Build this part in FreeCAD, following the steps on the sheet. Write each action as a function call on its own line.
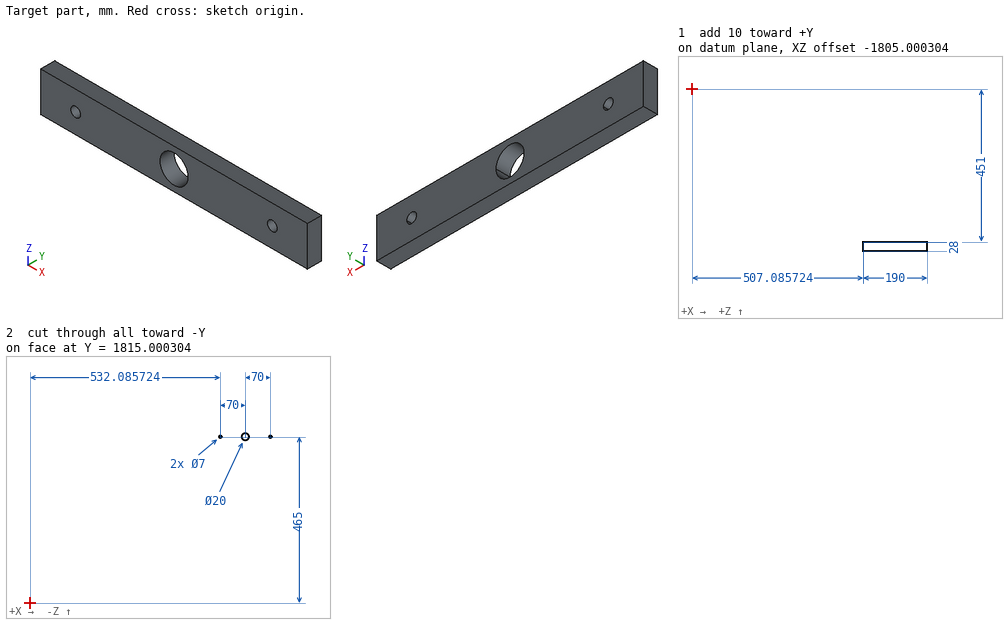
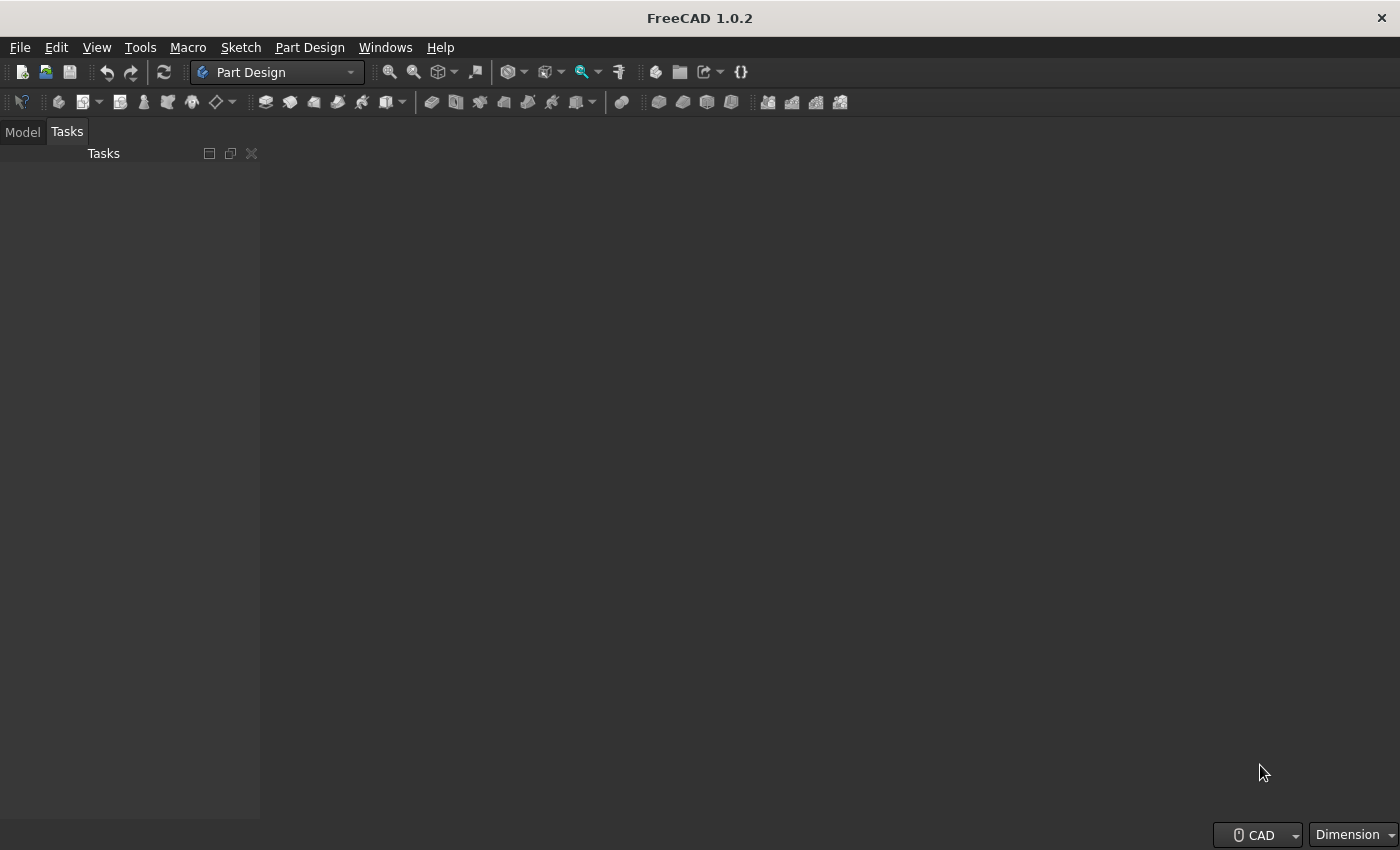
click(22, 72)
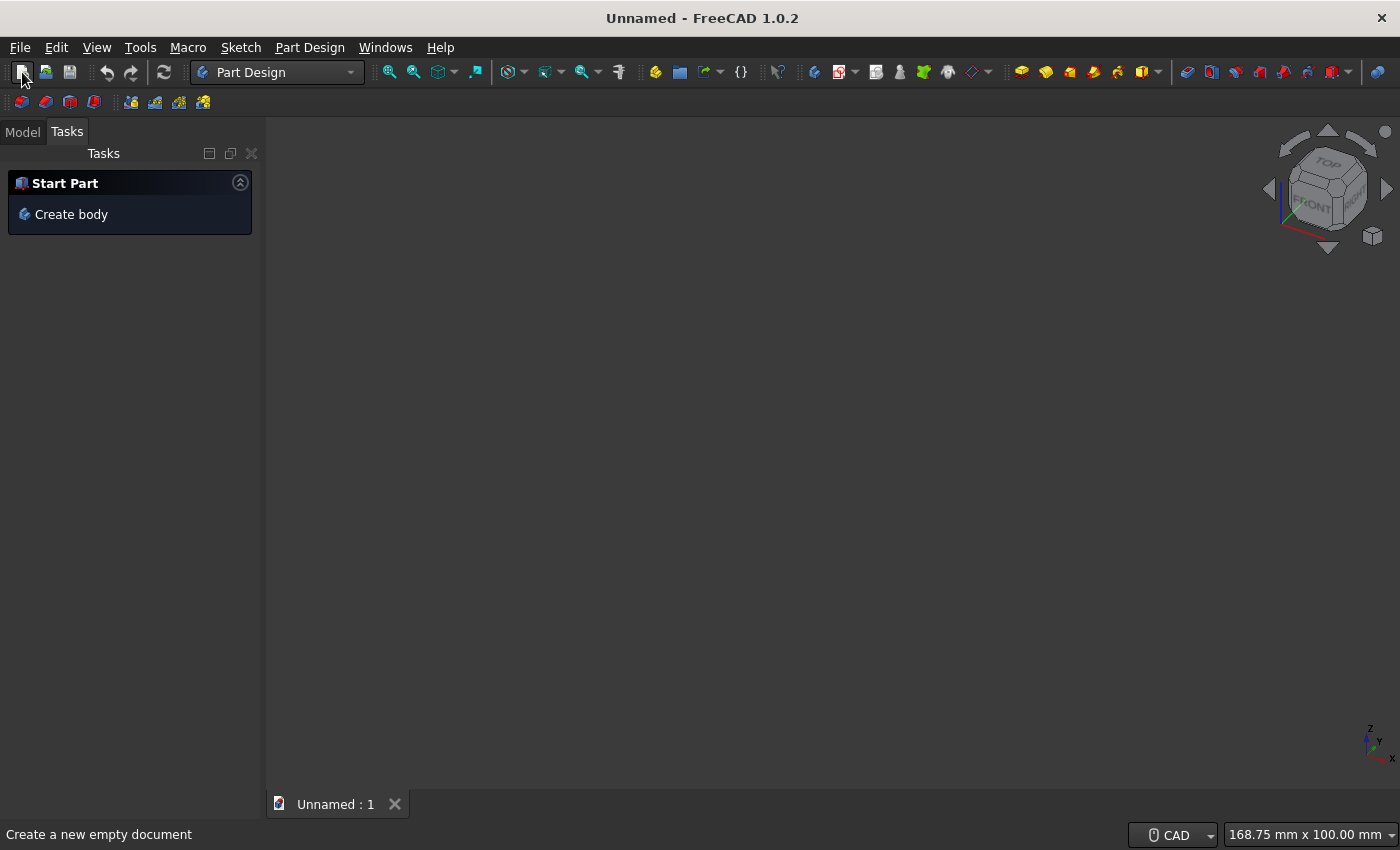
click(816, 72)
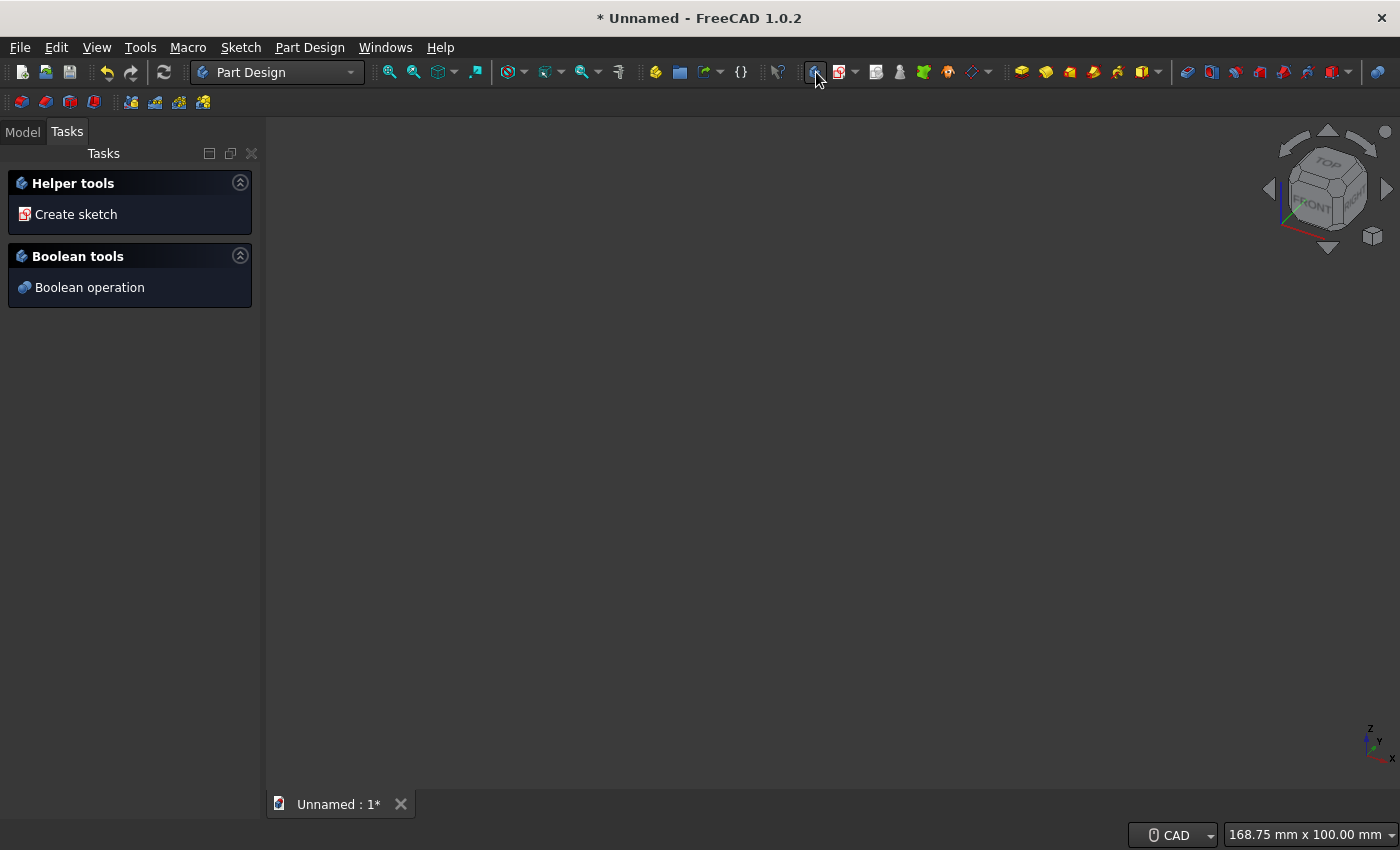
click(23, 131)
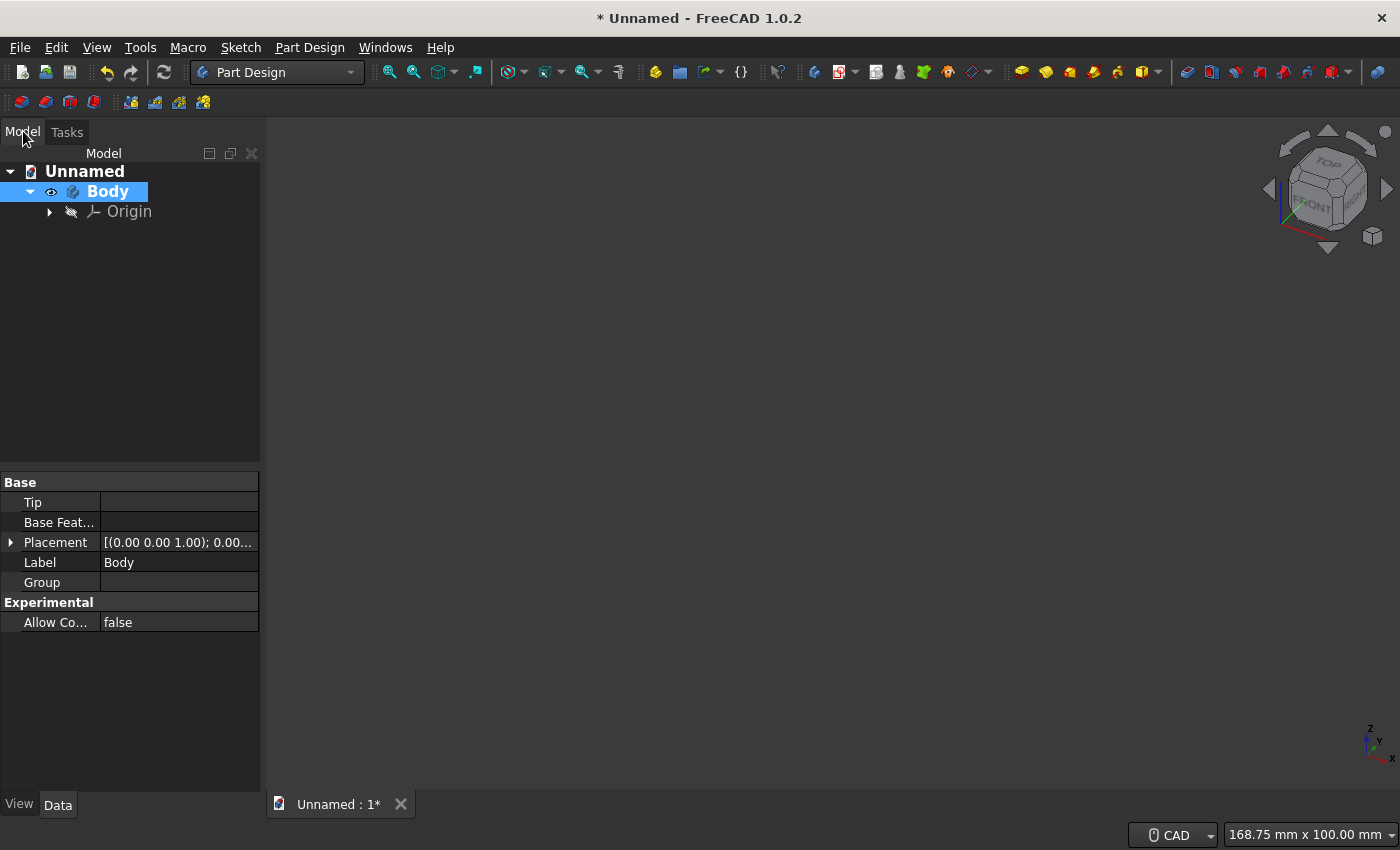
click(50, 212)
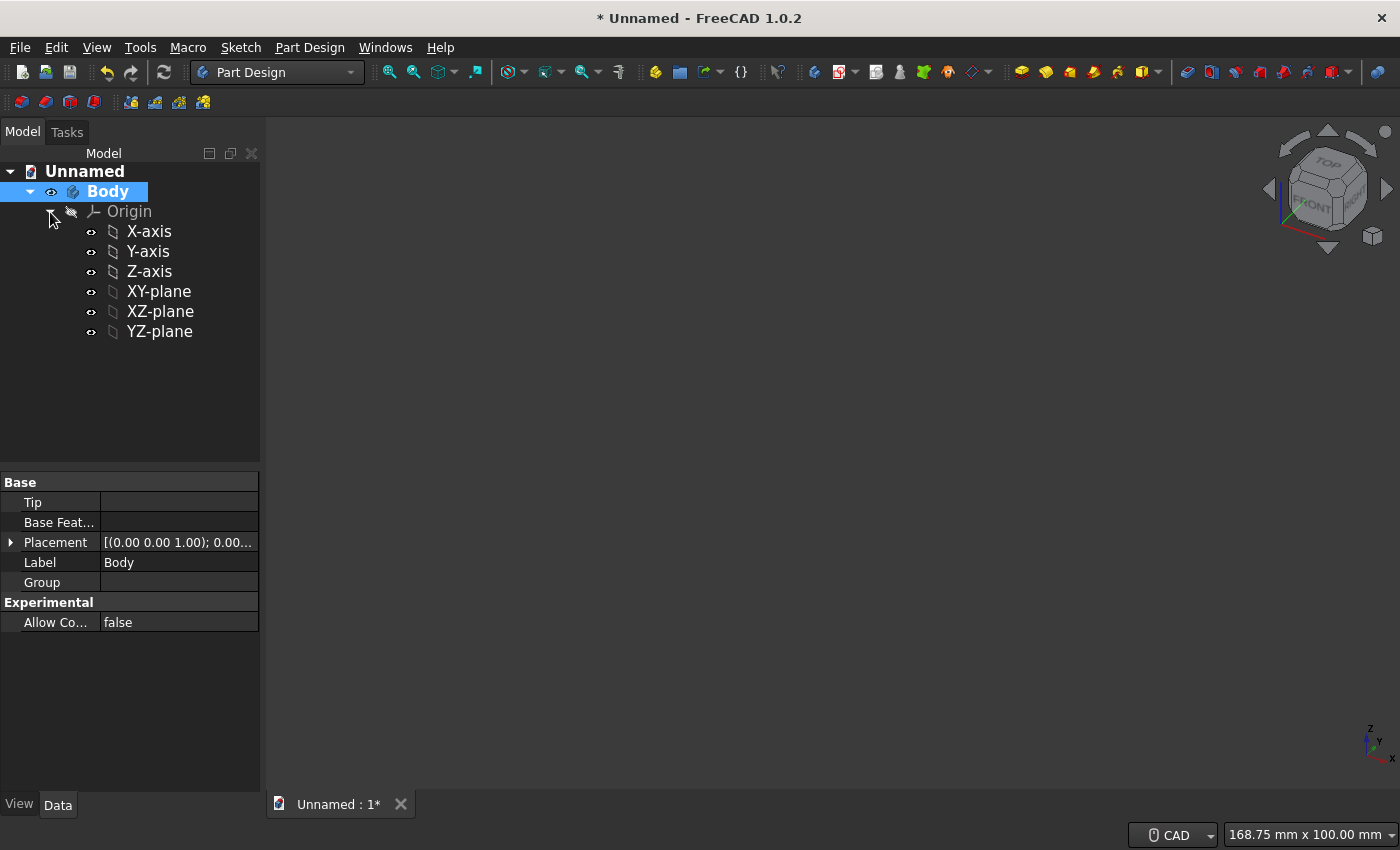
click(136, 312)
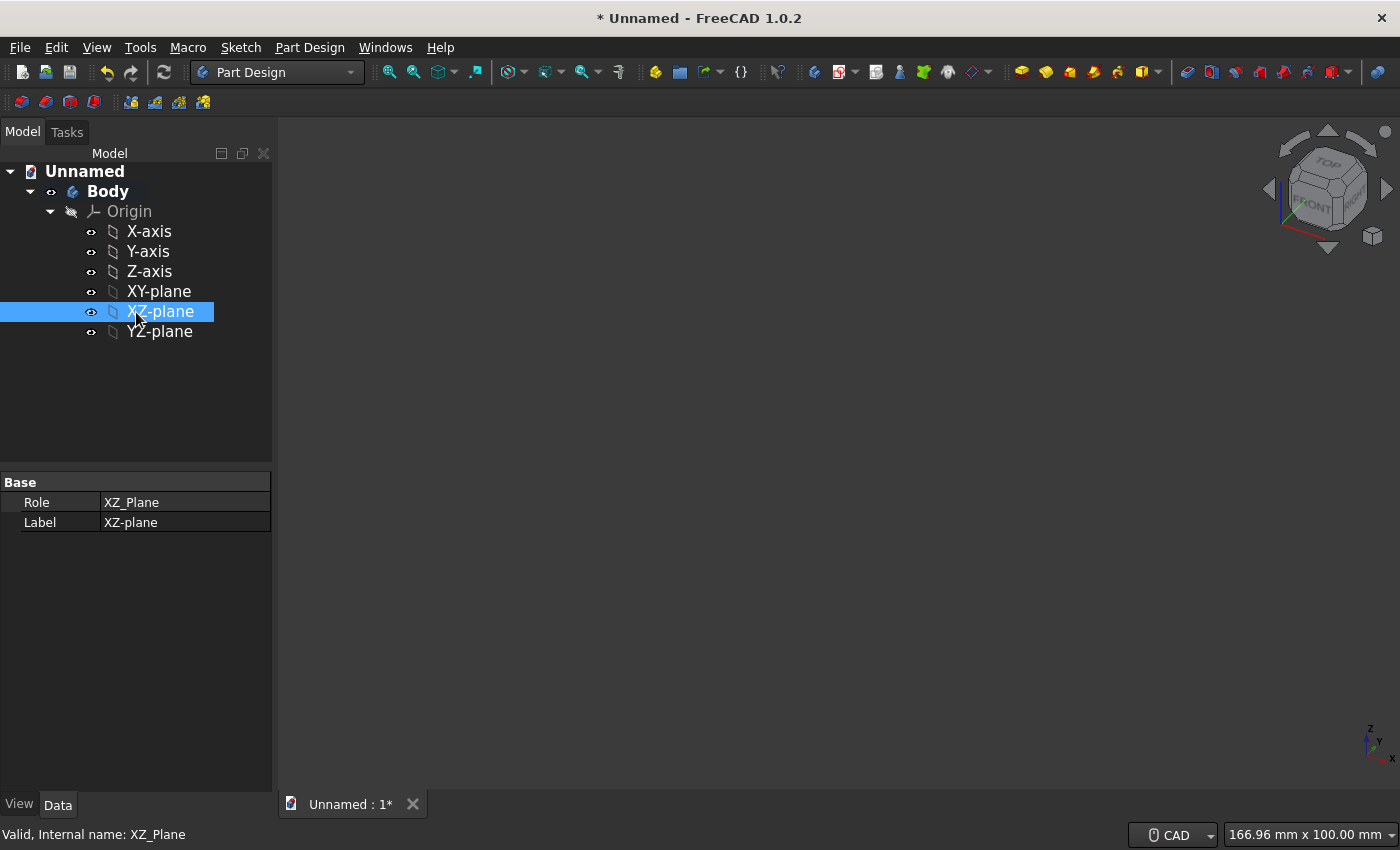
click(972, 72)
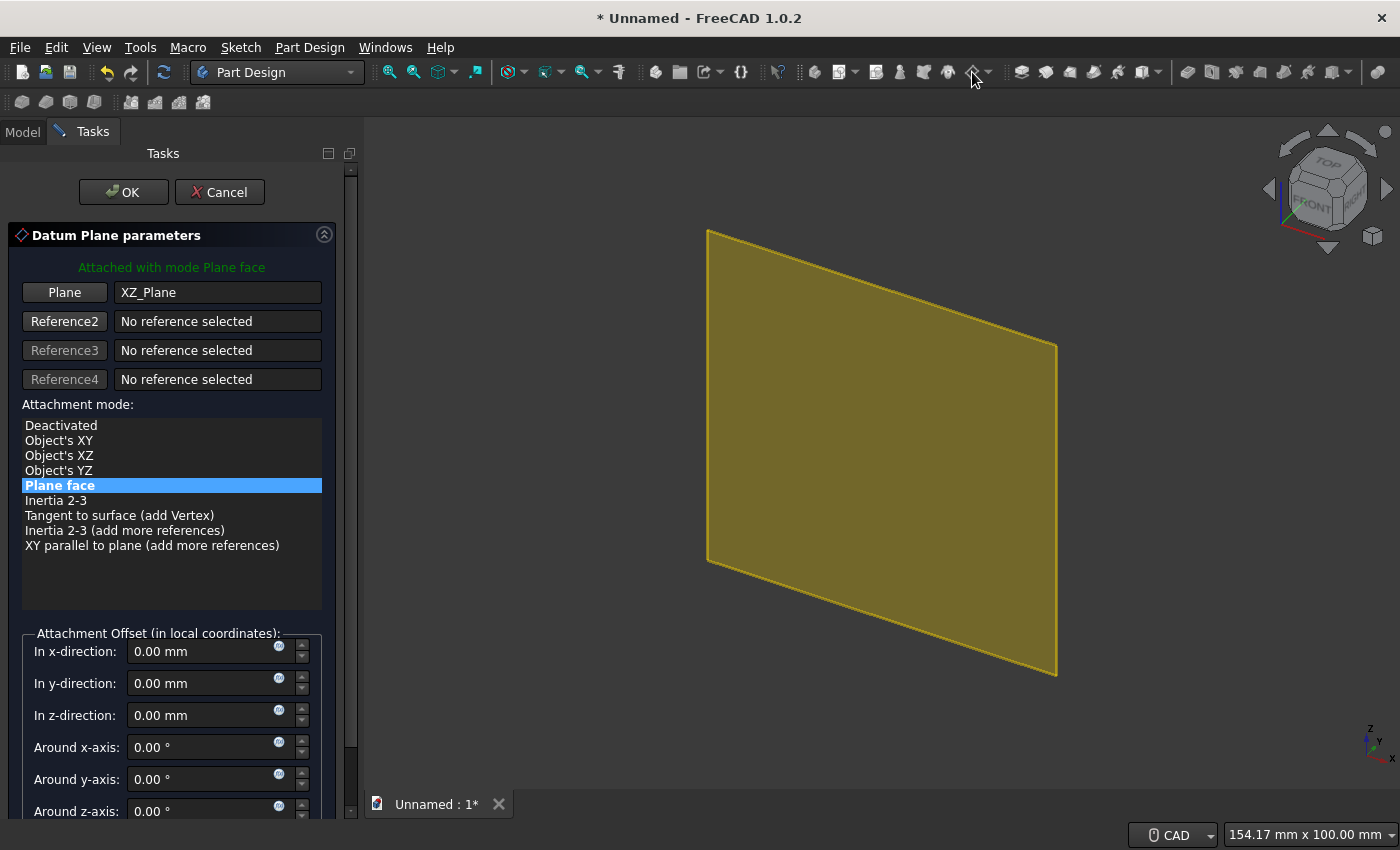
triple_click(210, 715)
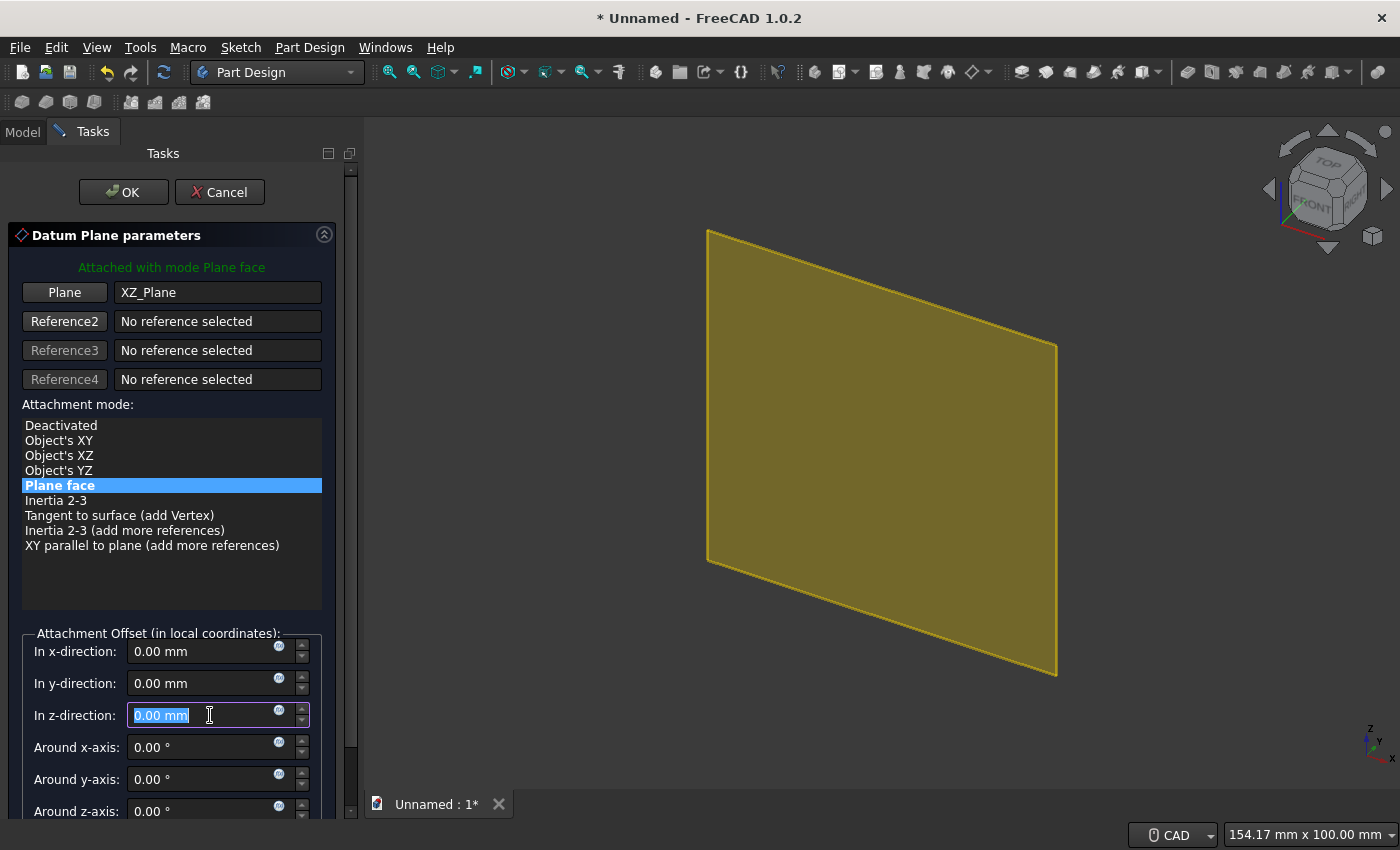
text(-1805.000304)
key(Tab)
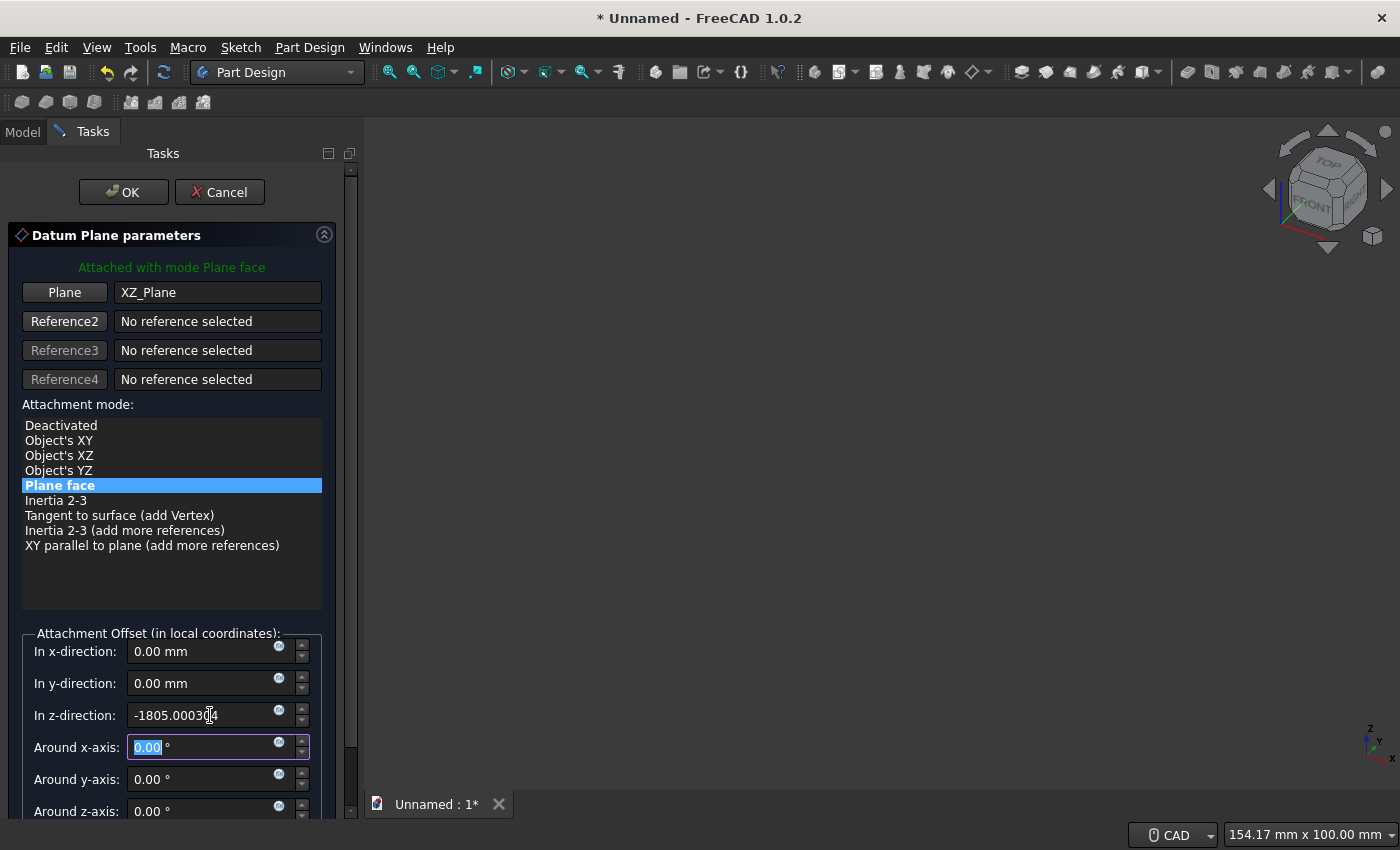
click(124, 192)